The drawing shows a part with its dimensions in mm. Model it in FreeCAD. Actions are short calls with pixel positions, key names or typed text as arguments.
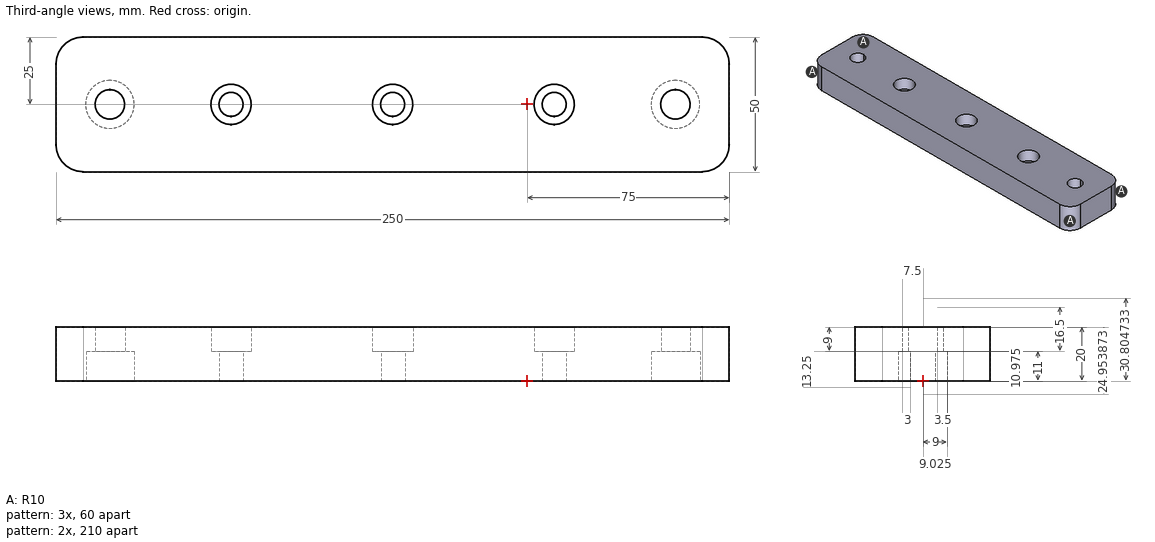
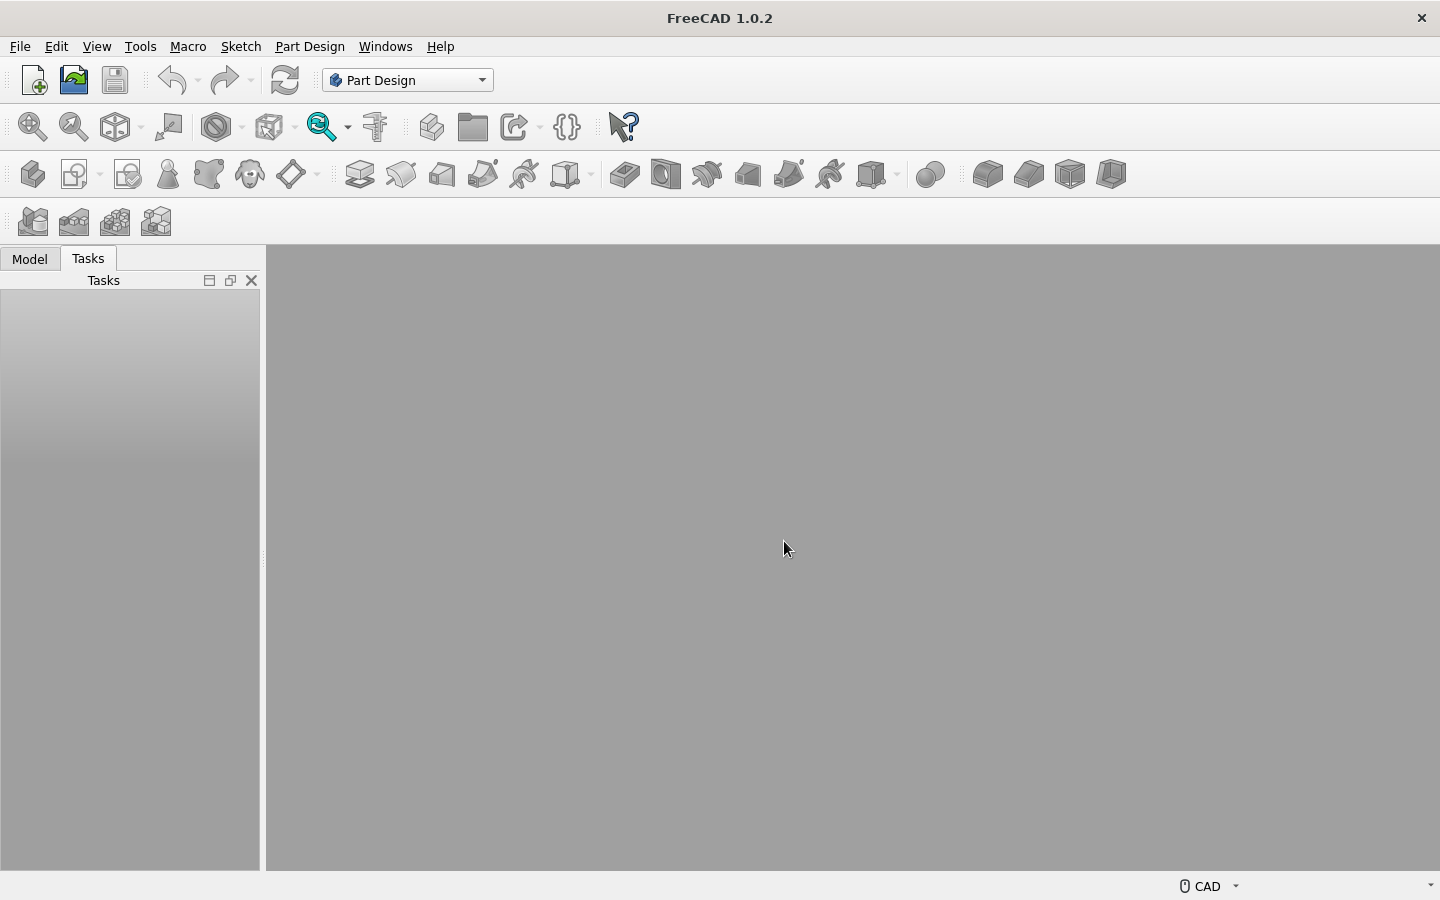
click(33, 80)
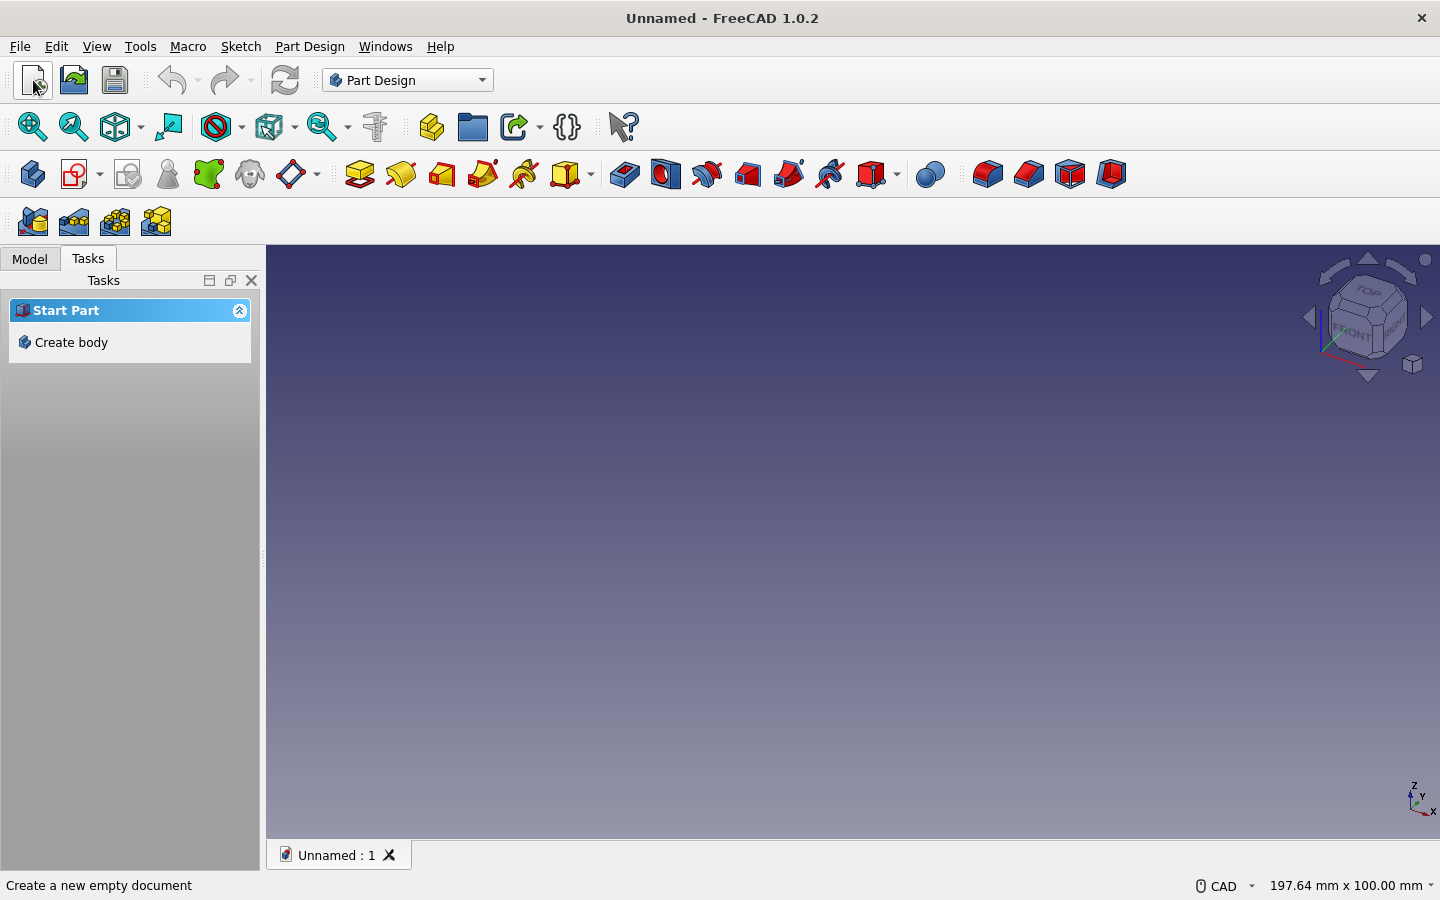
click(74, 174)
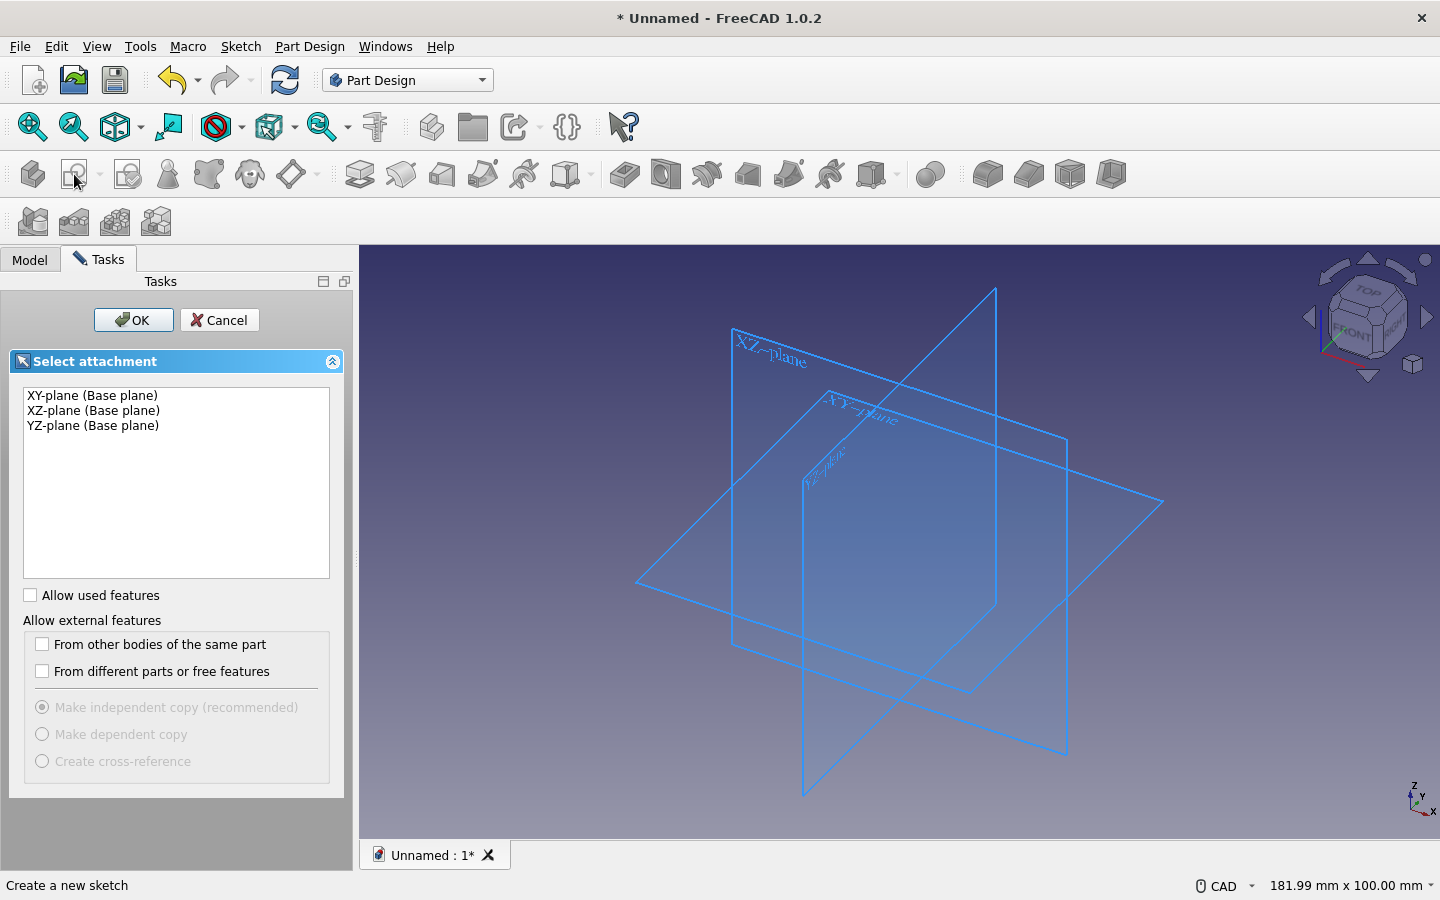
click(84, 396)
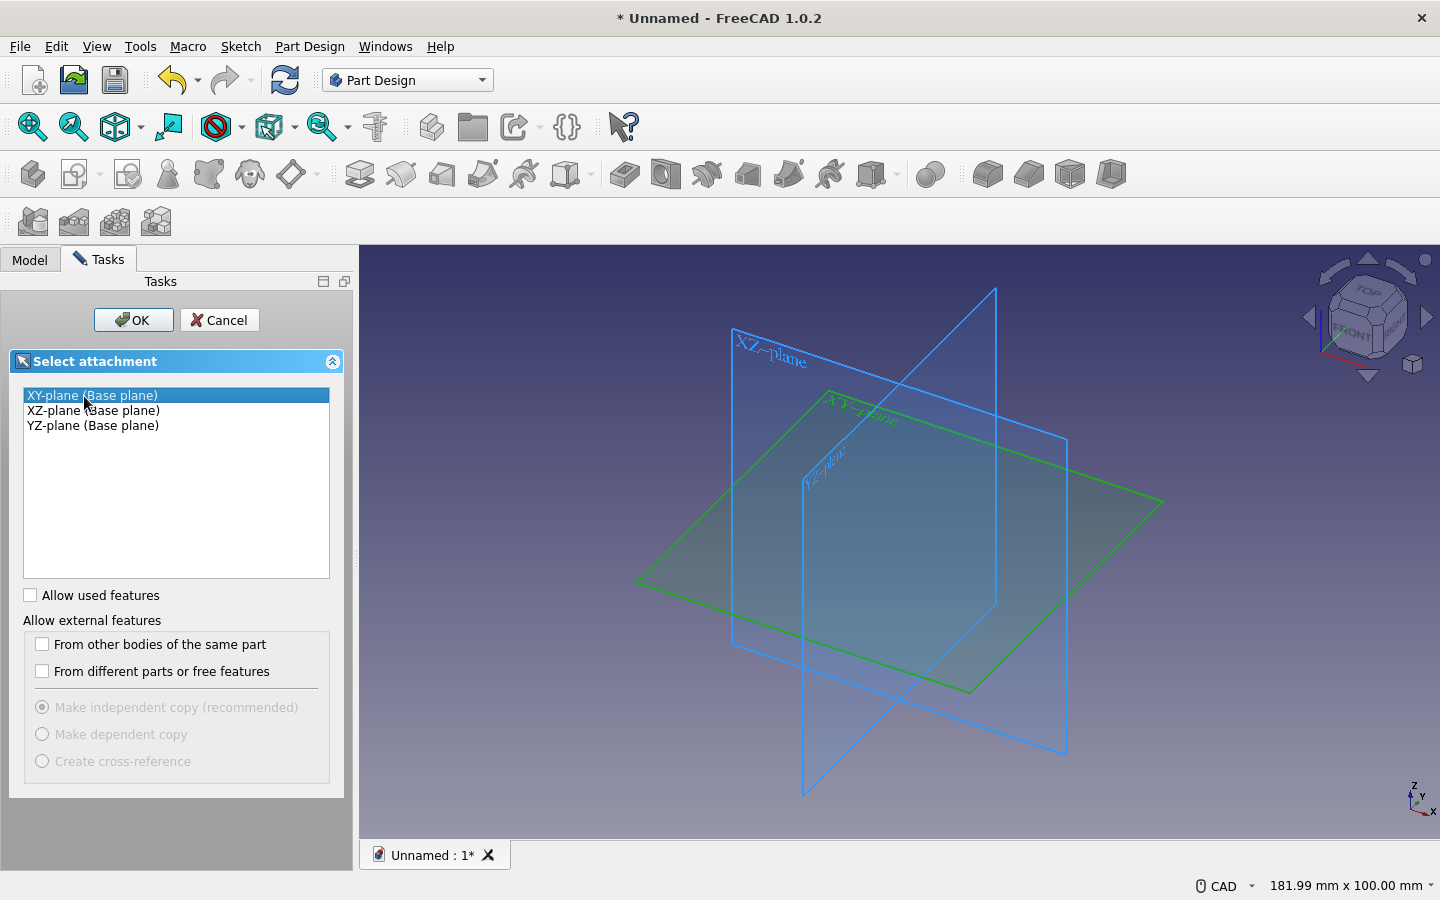
click(134, 320)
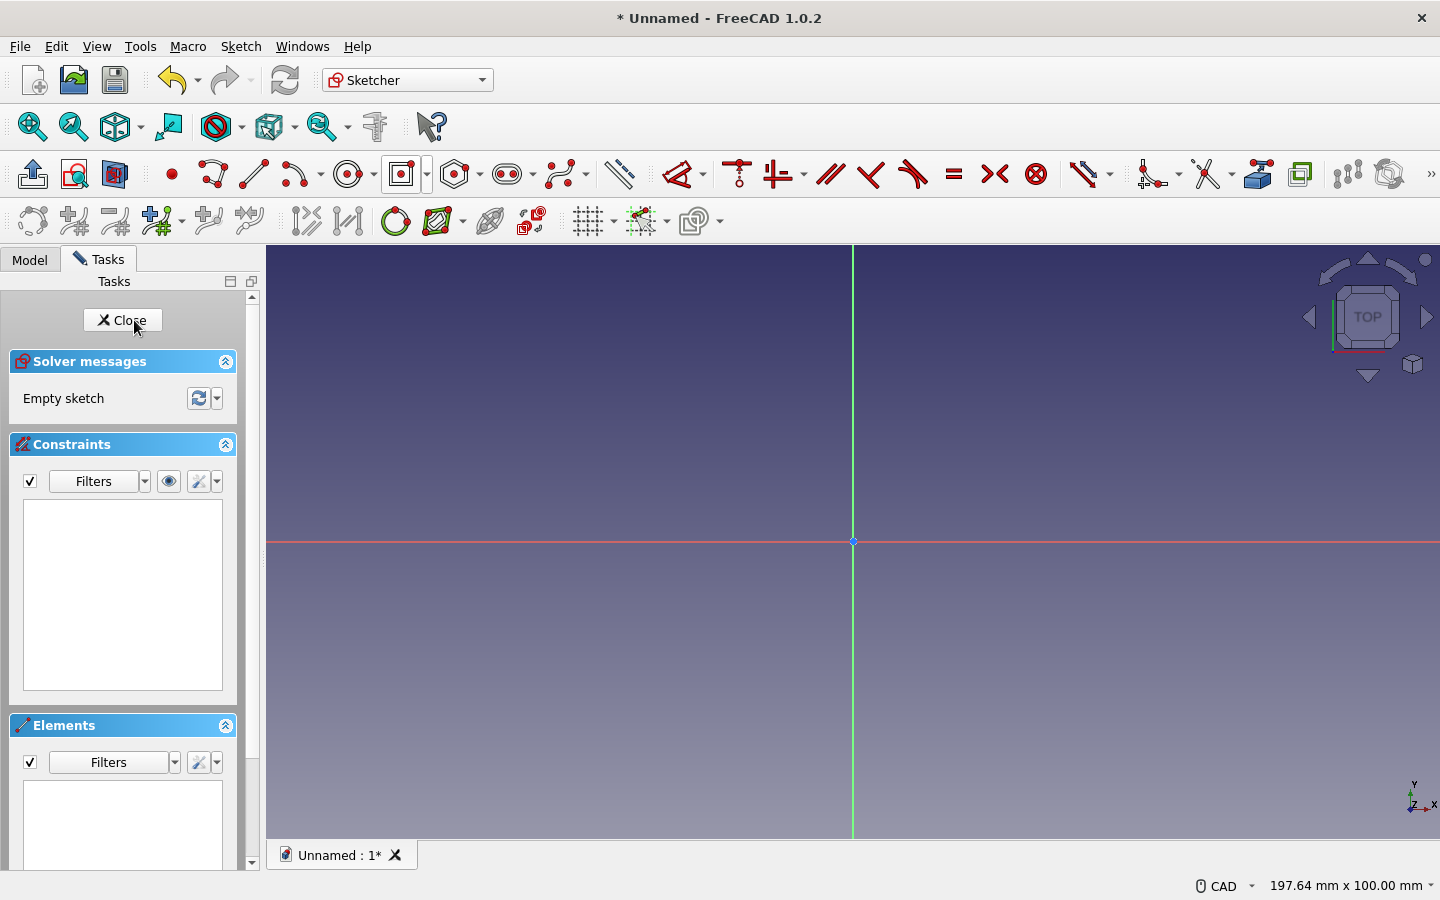
scroll(971, 542, down, 4)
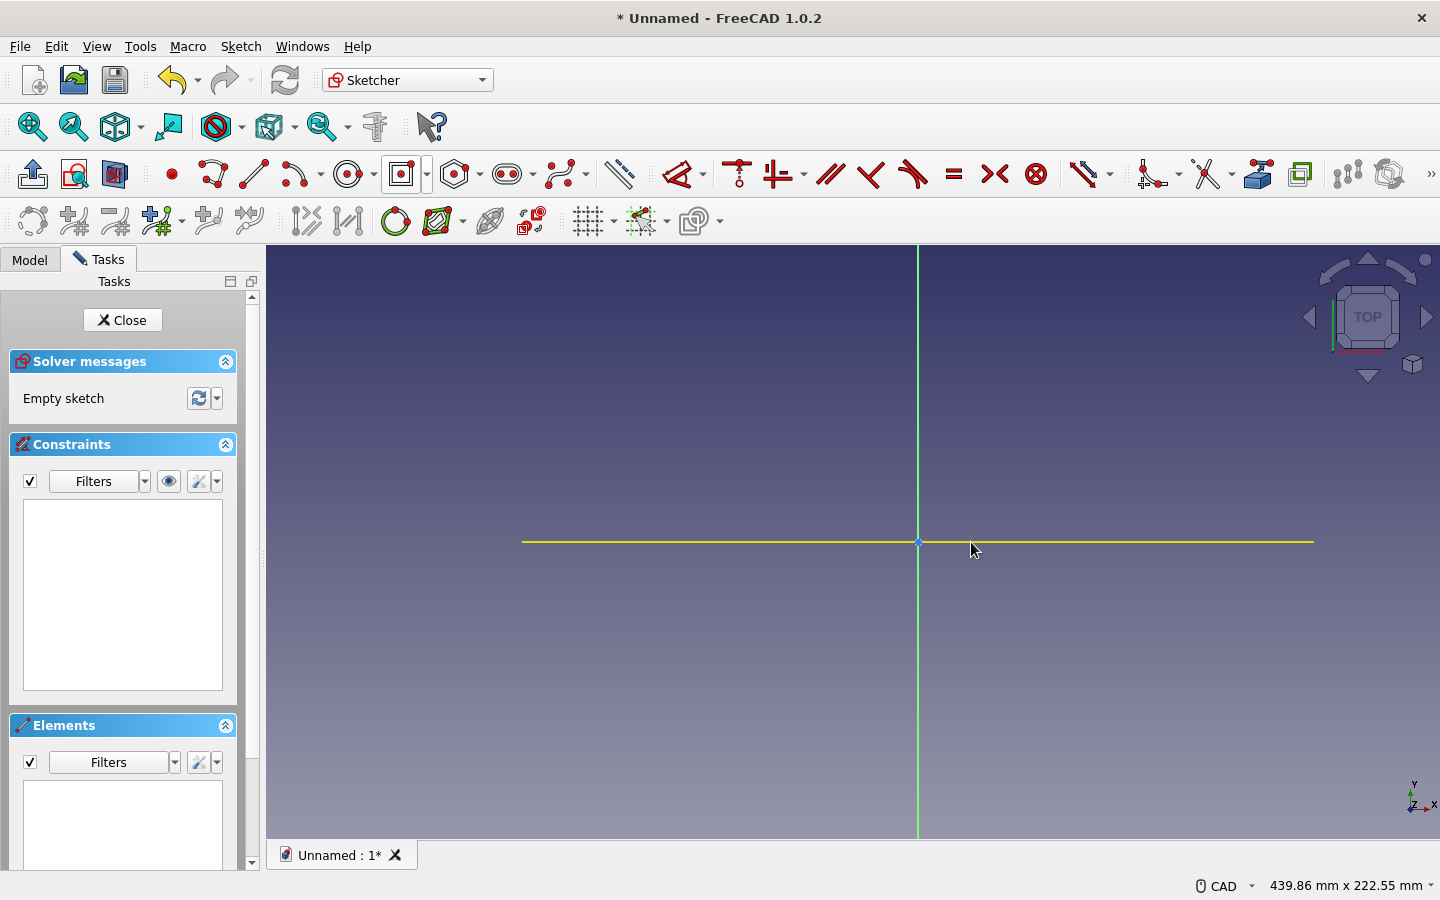
key(g)
key(r)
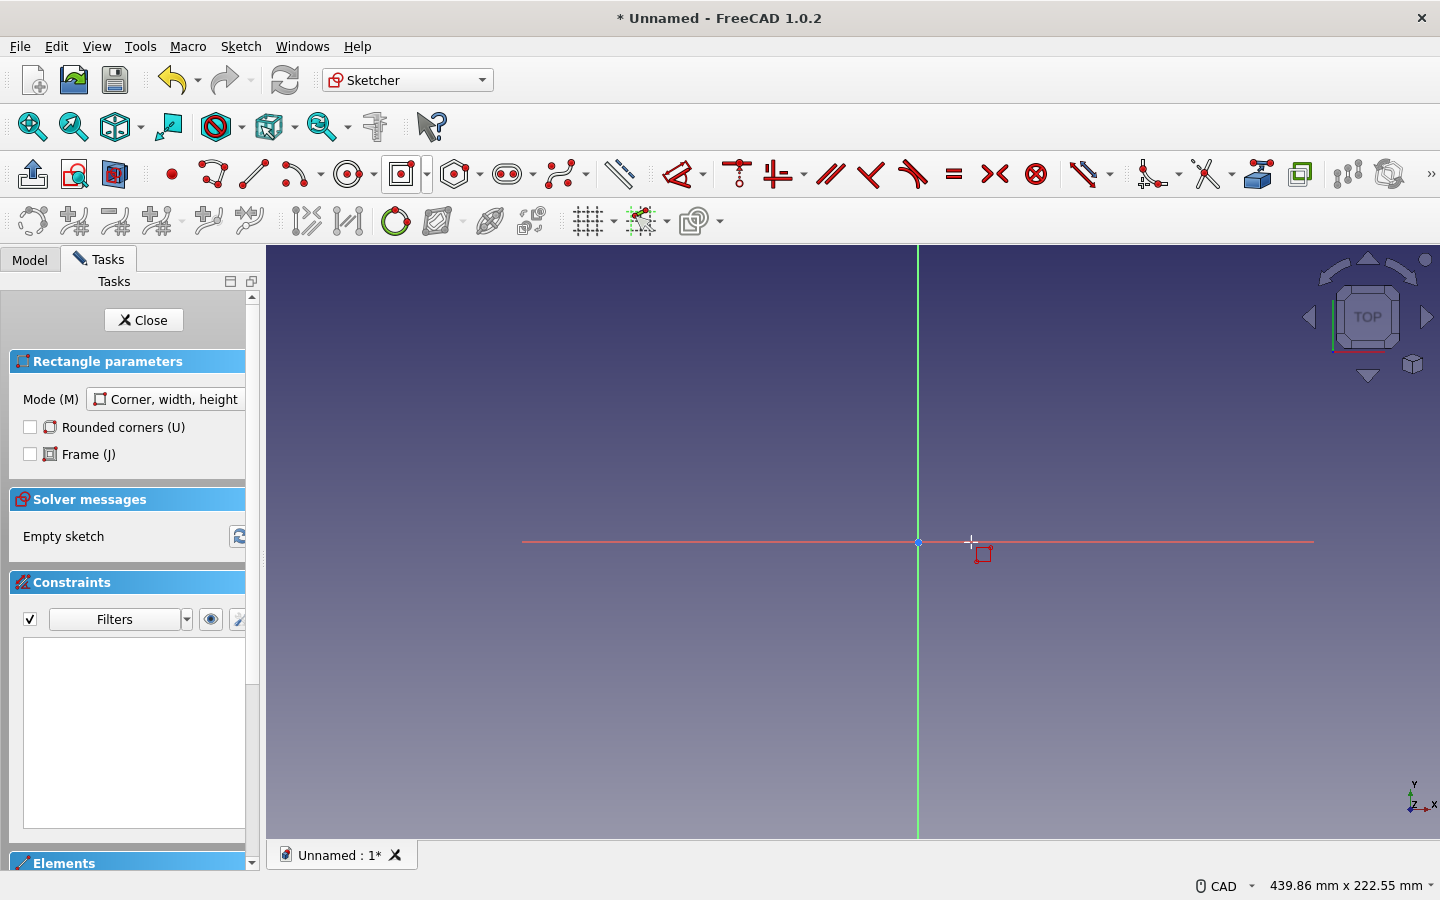
click(451, 476)
move(1118, 609)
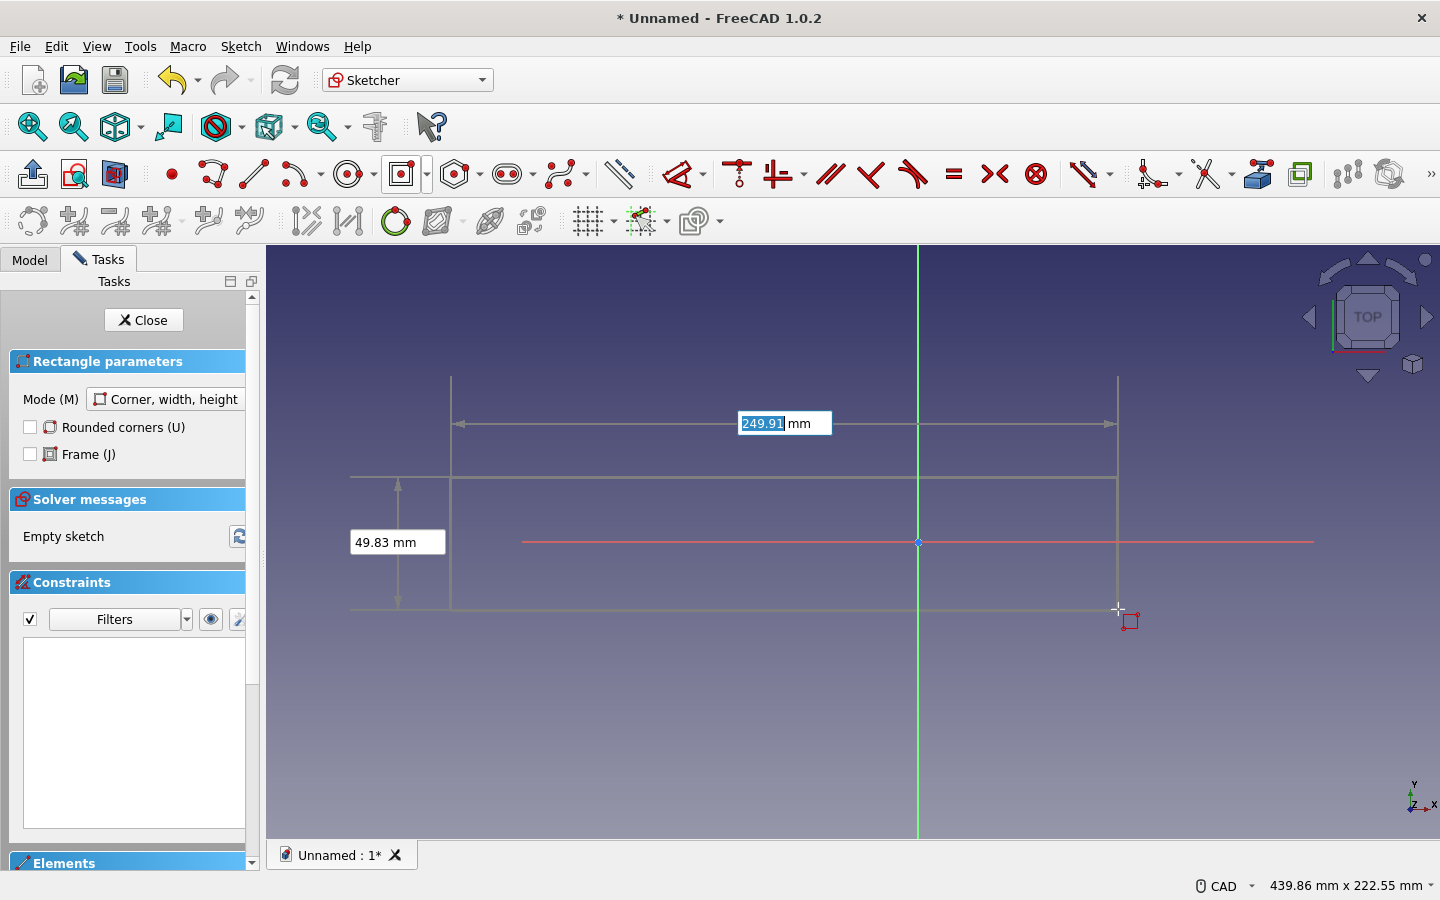
text(250)
key(Tab)
text(50)
key(Return)
key(Escape)